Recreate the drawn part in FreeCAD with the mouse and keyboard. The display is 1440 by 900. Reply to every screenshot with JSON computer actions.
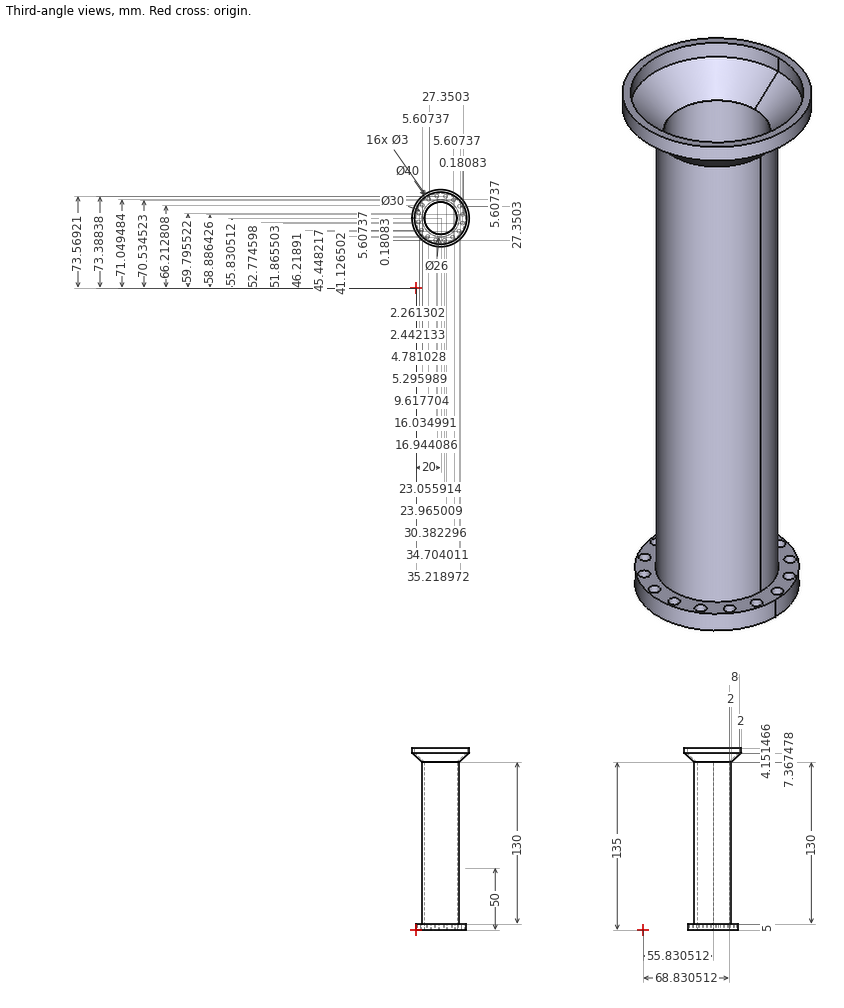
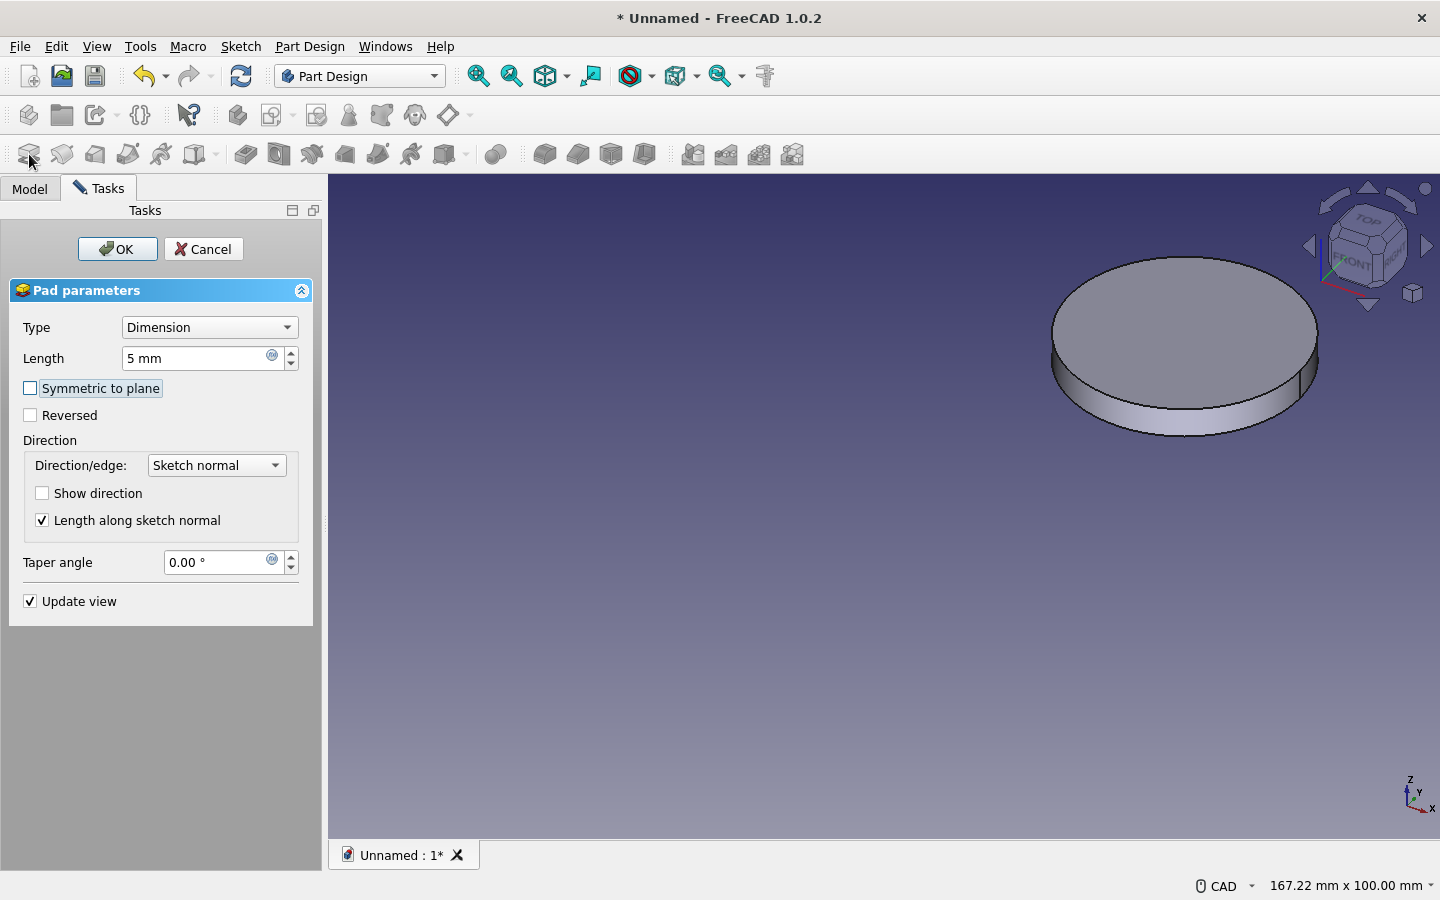
{"action": "left_click", "coordinate": [118, 249]}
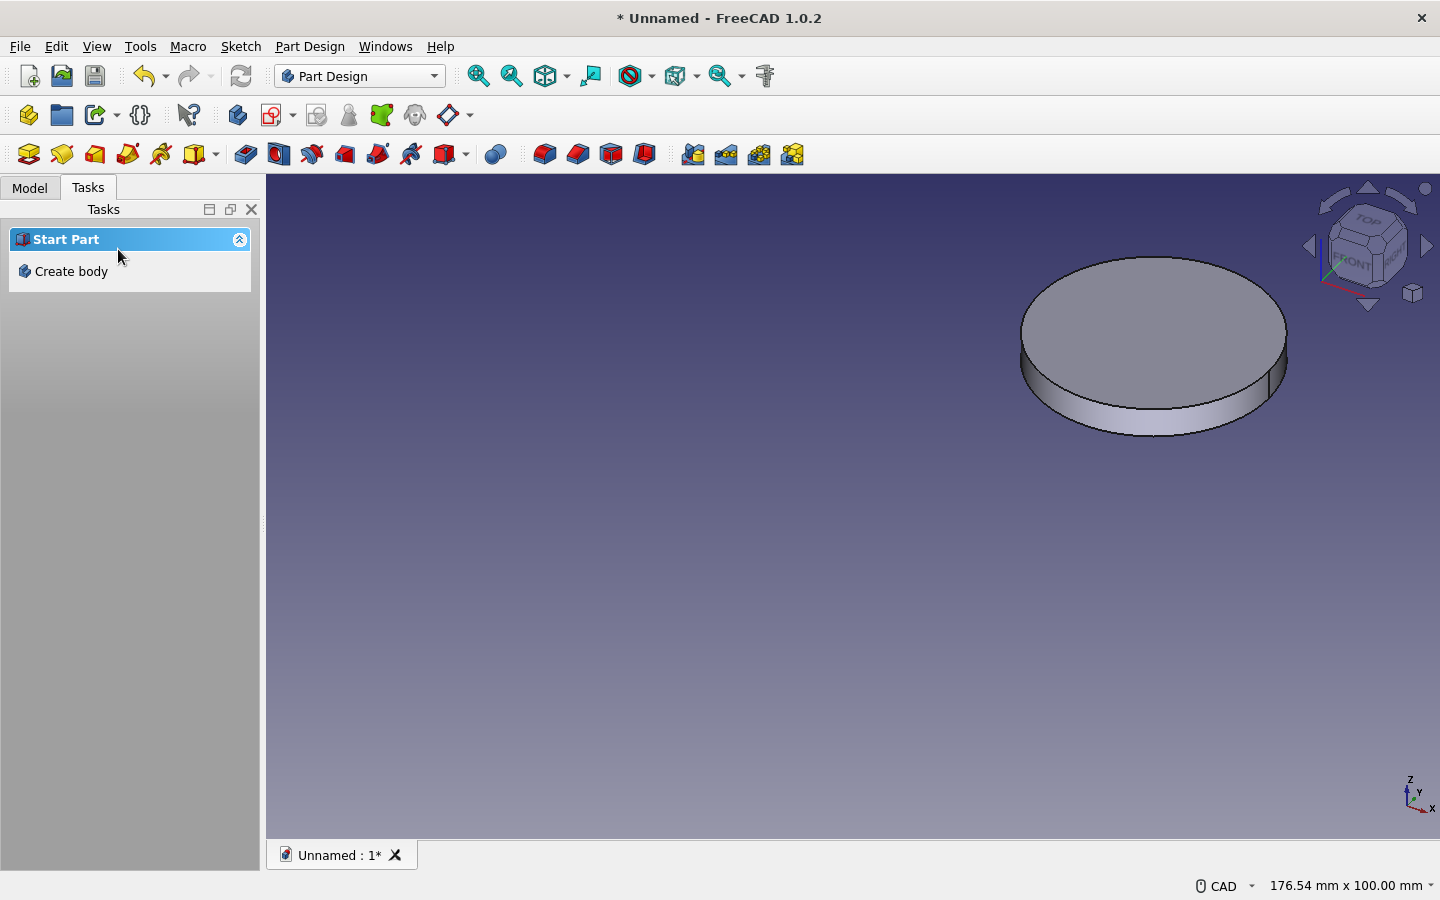
{"action": "key", "text": "v f"}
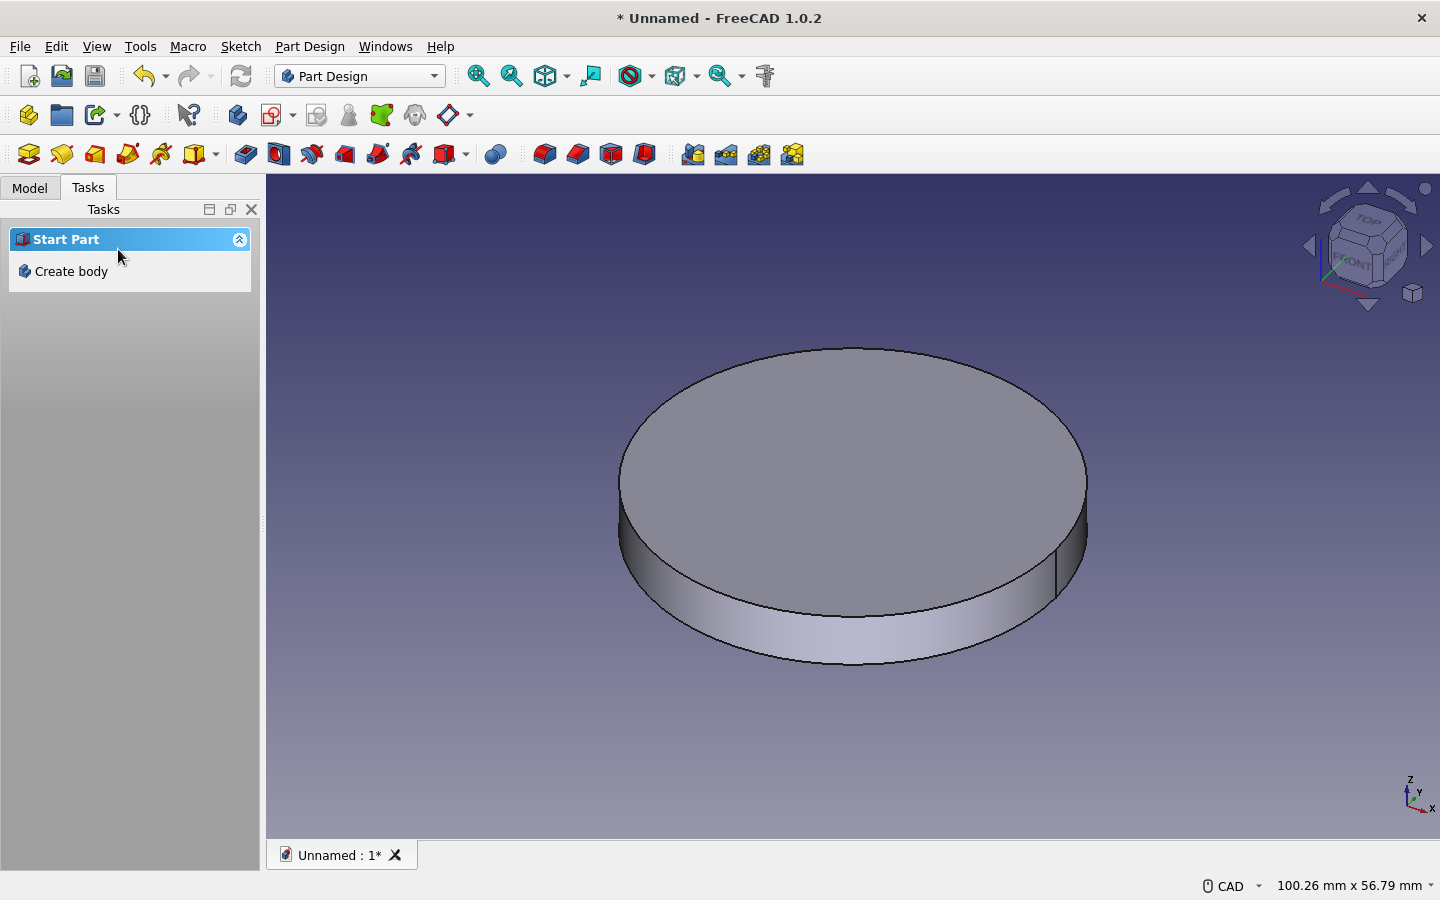
{"action": "left_click", "coordinate": [853, 482]}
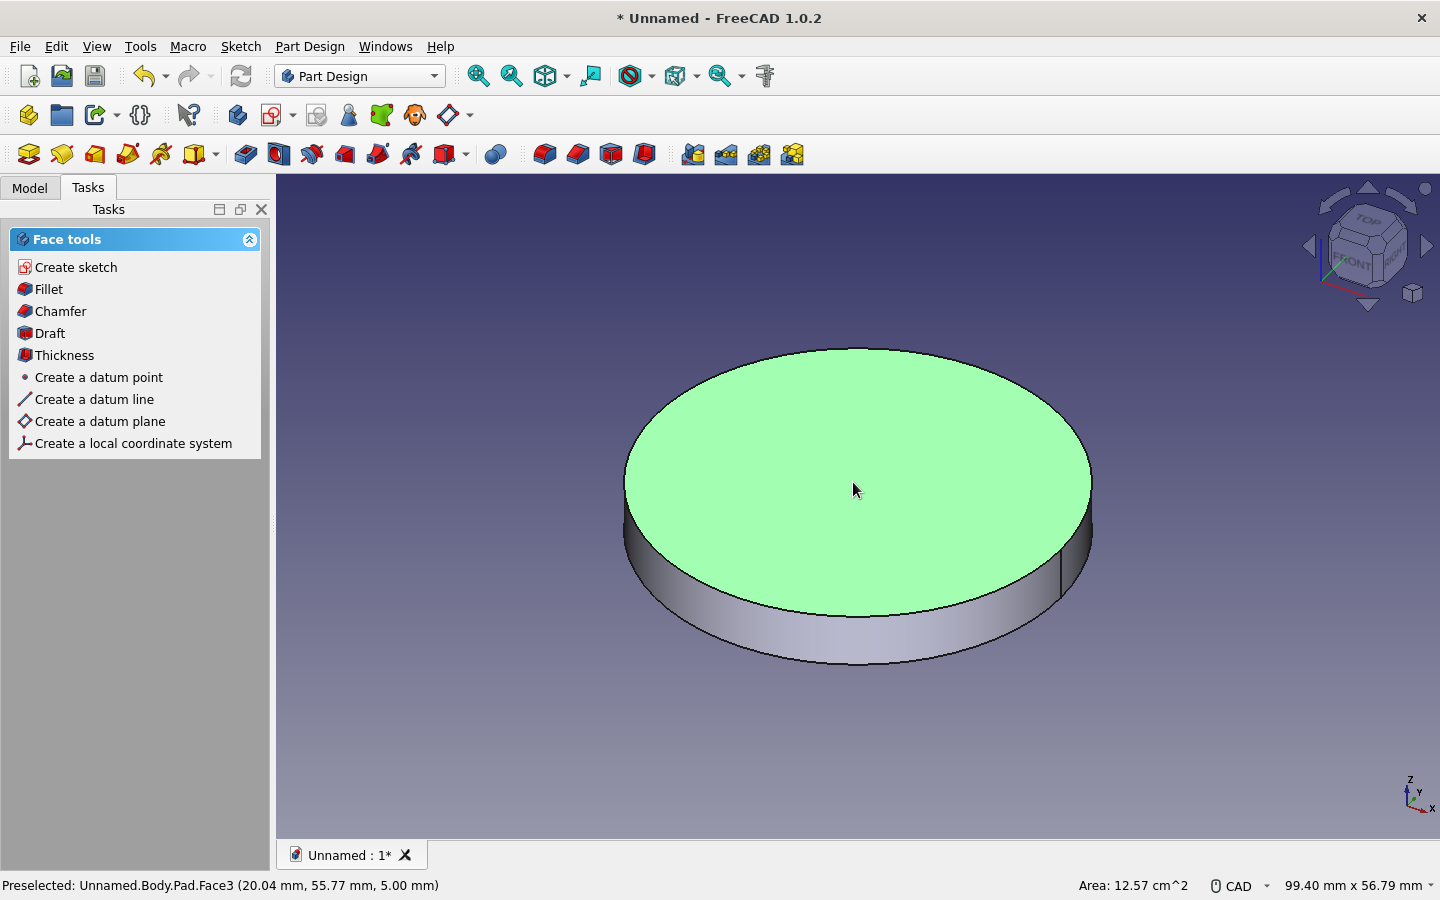
{"action": "left_click", "coordinate": [270, 116]}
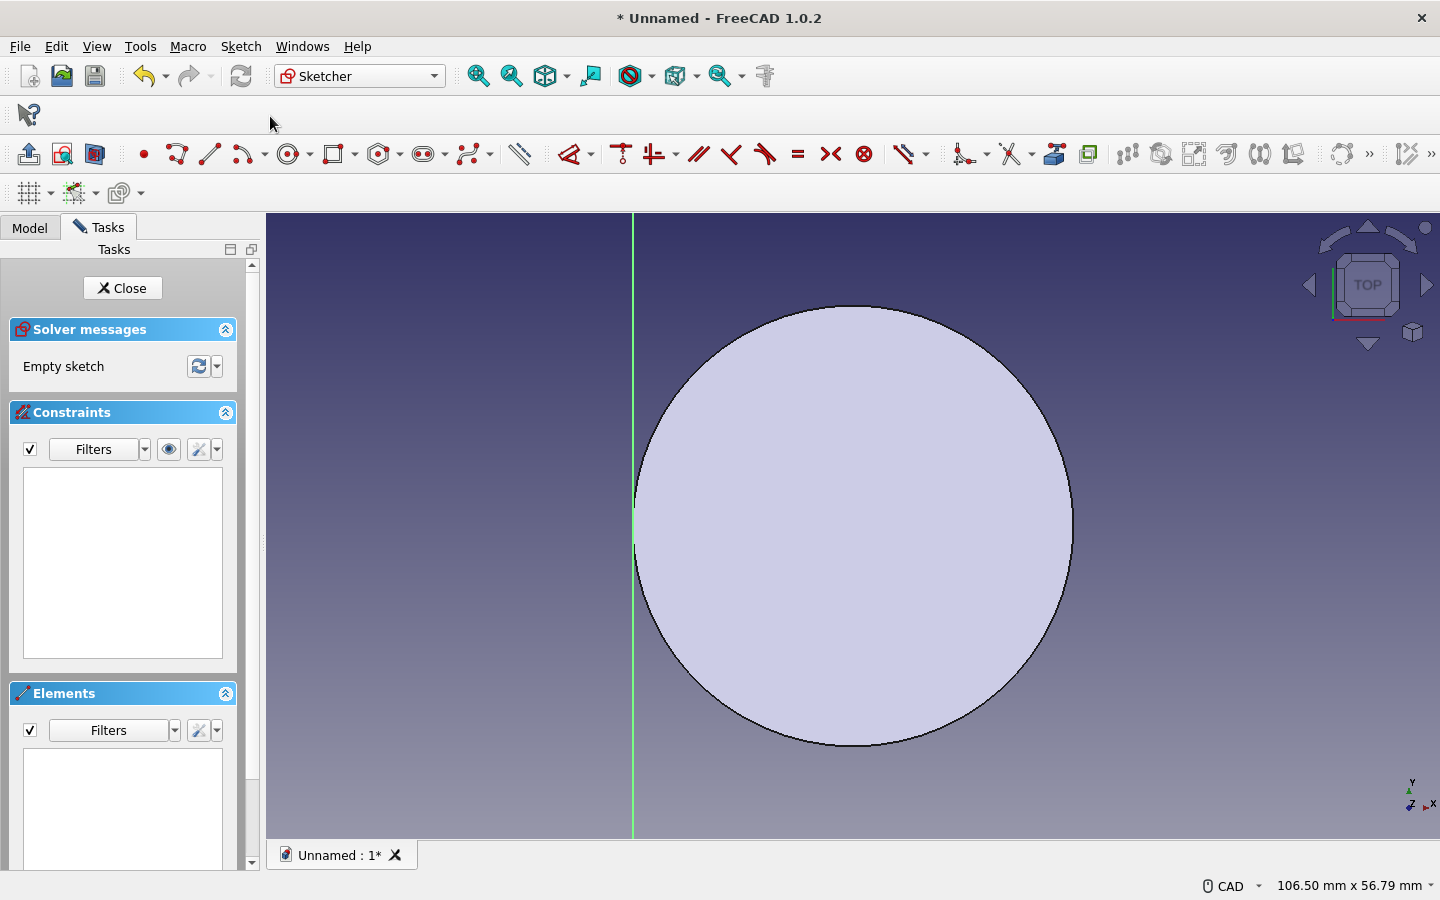
{"action": "scroll", "coordinate": [735, 252], "scroll_direction": "down", "scroll_amount": 3}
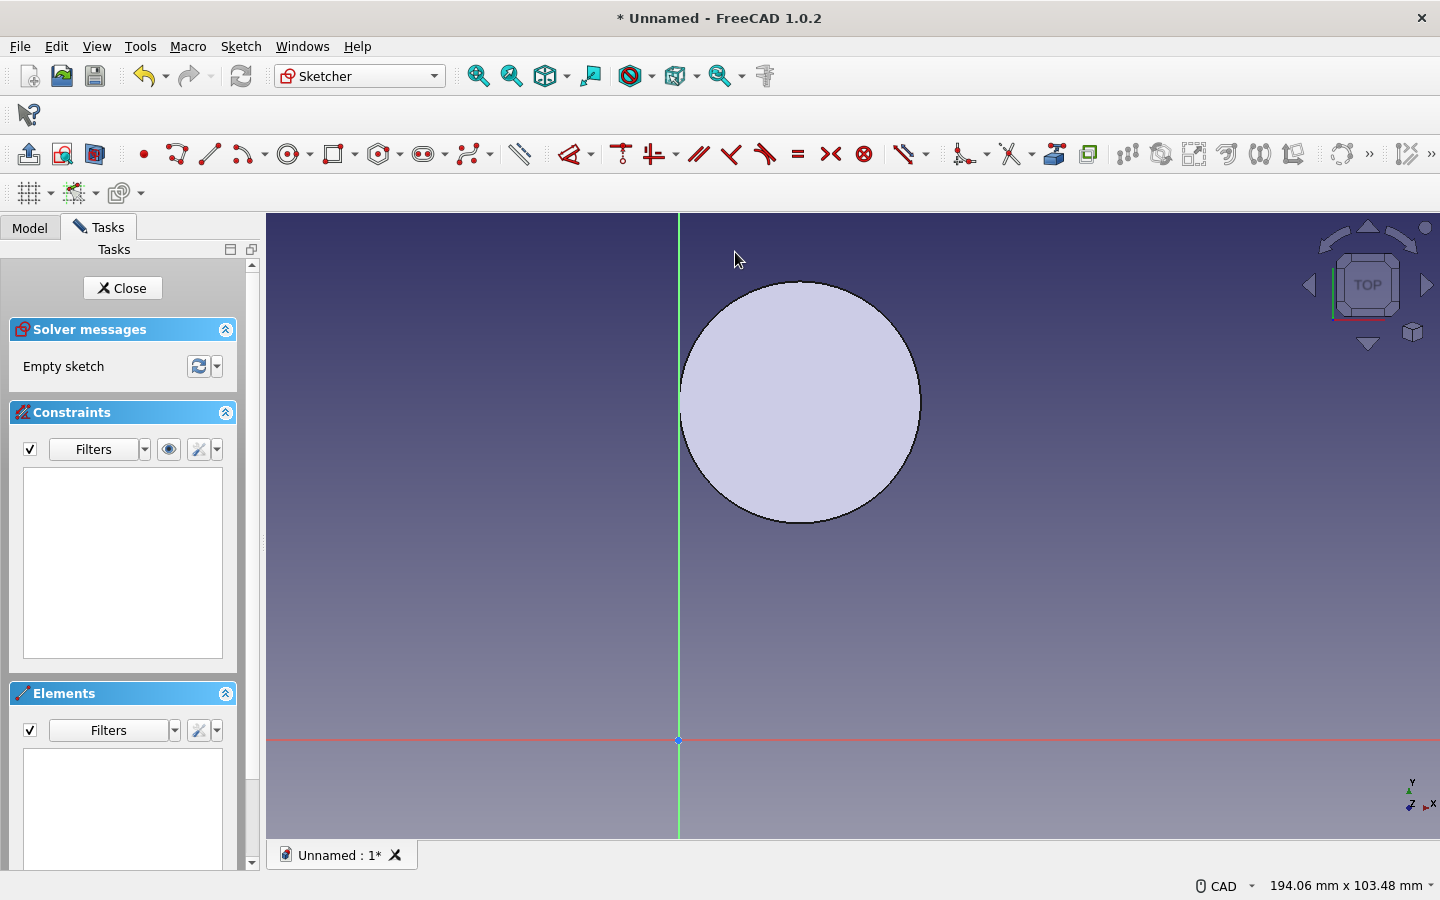
{"action": "left_click", "coordinate": [288, 154]}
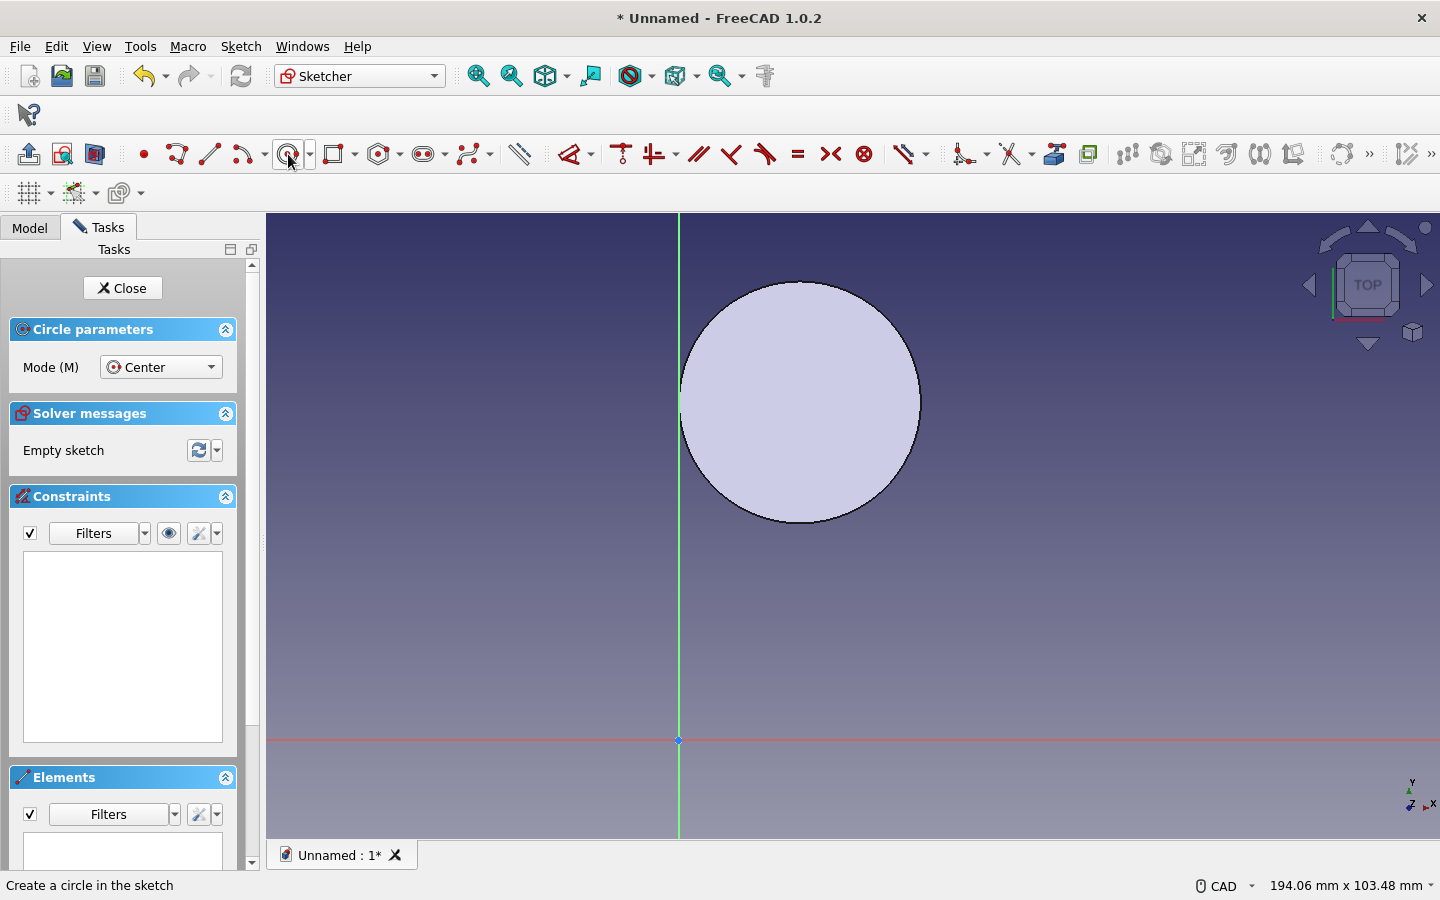
{"action": "left_click", "coordinate": [800, 402]}
{"action": "mouse_move", "coordinate": [864, 338]}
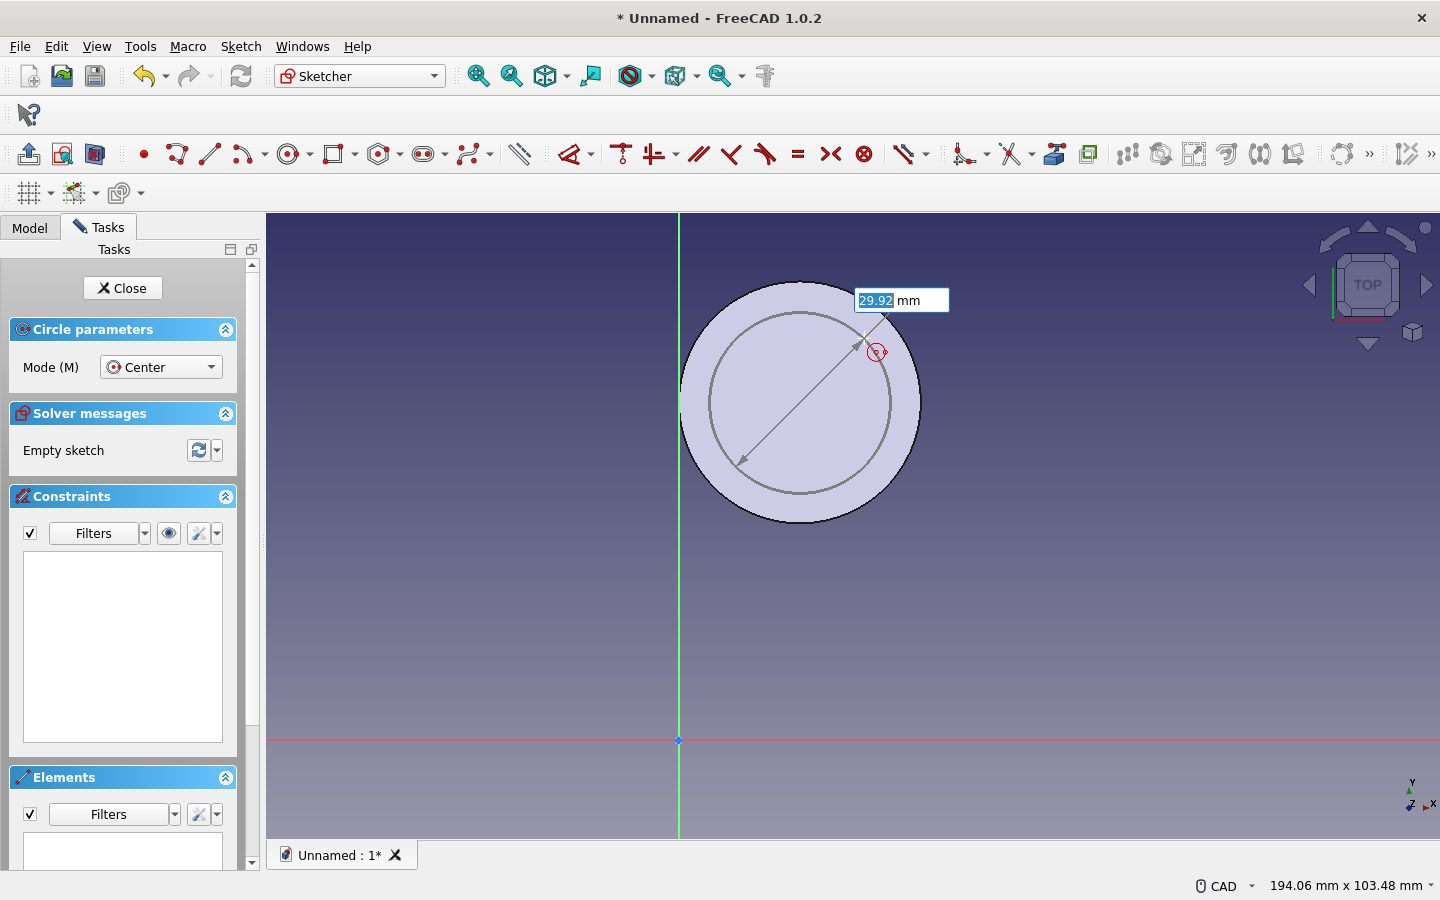
{"action": "type", "text": "30"}
{"action": "key", "text": "Return"}
{"action": "key", "text": "Escape"}